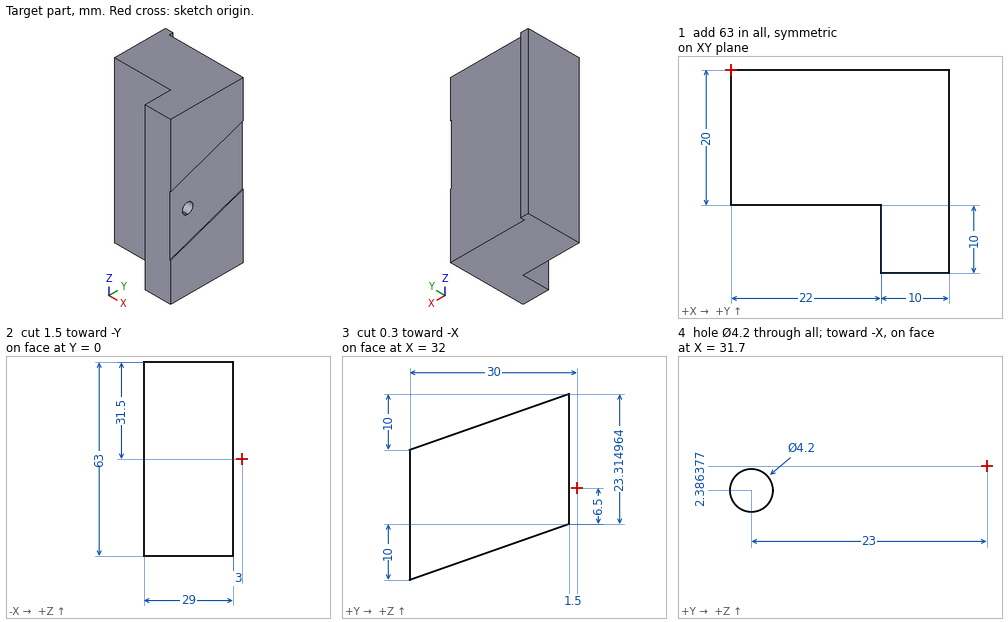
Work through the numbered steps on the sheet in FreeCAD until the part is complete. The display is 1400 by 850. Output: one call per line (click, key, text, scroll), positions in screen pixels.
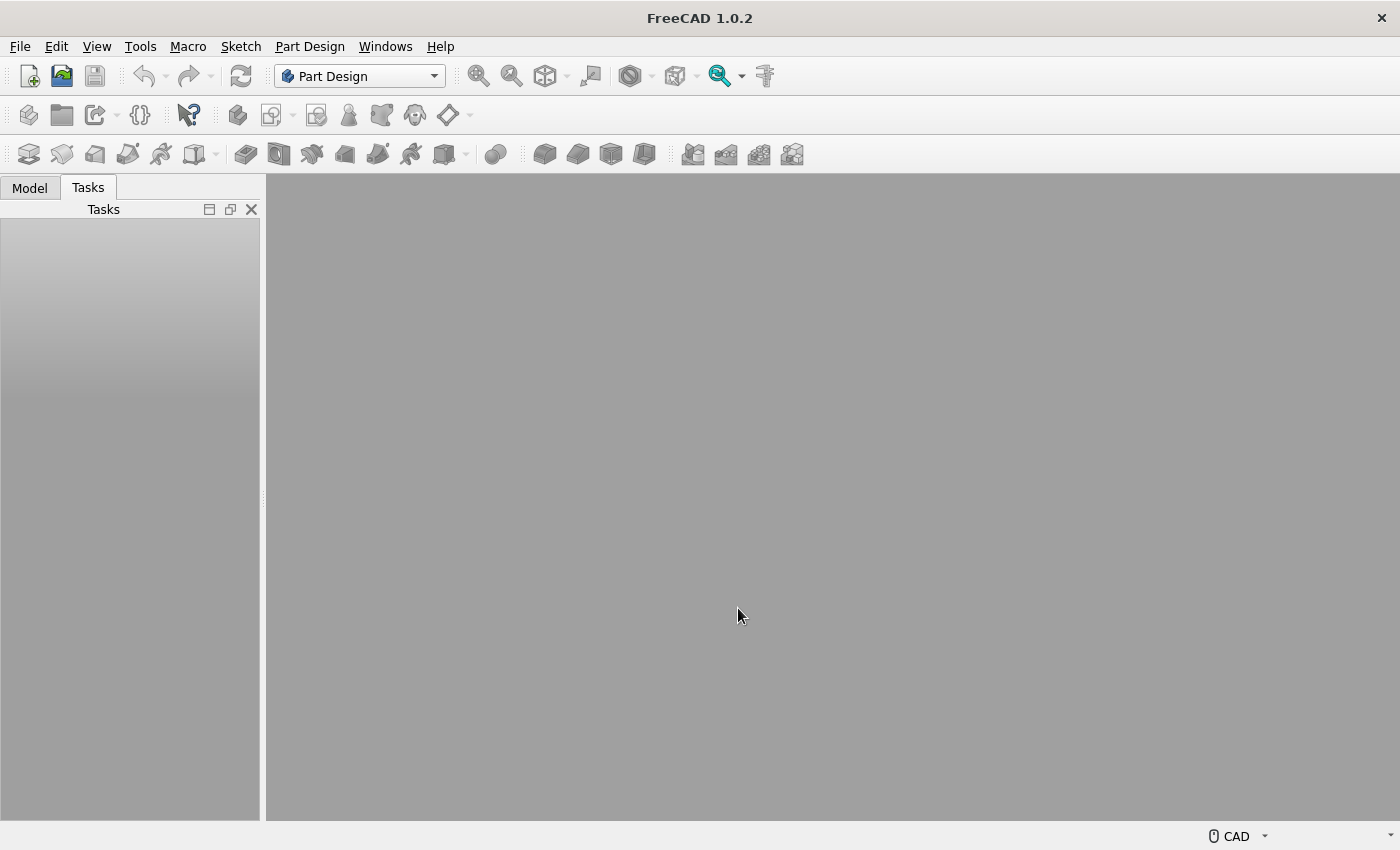
click(29, 76)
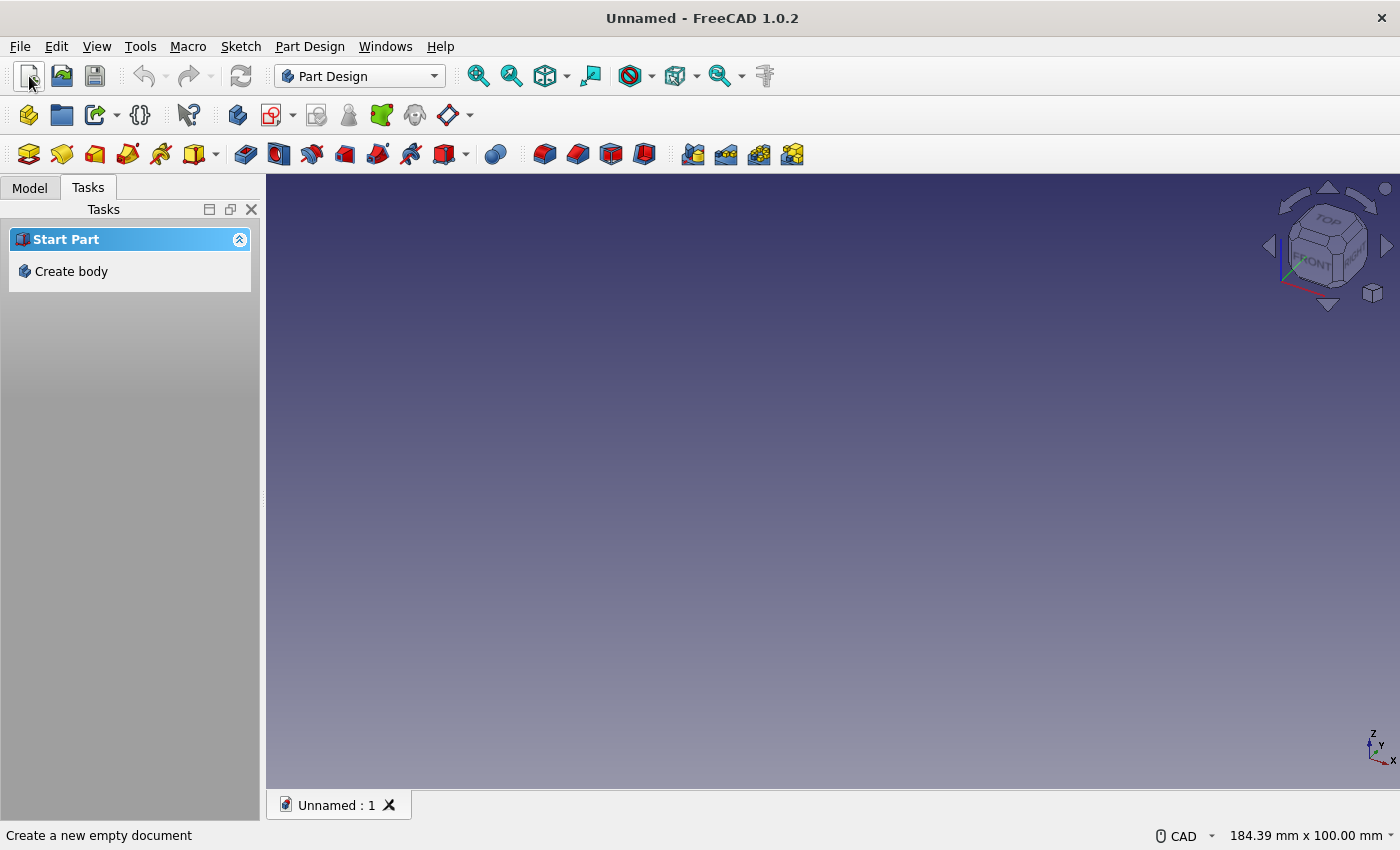
click(270, 116)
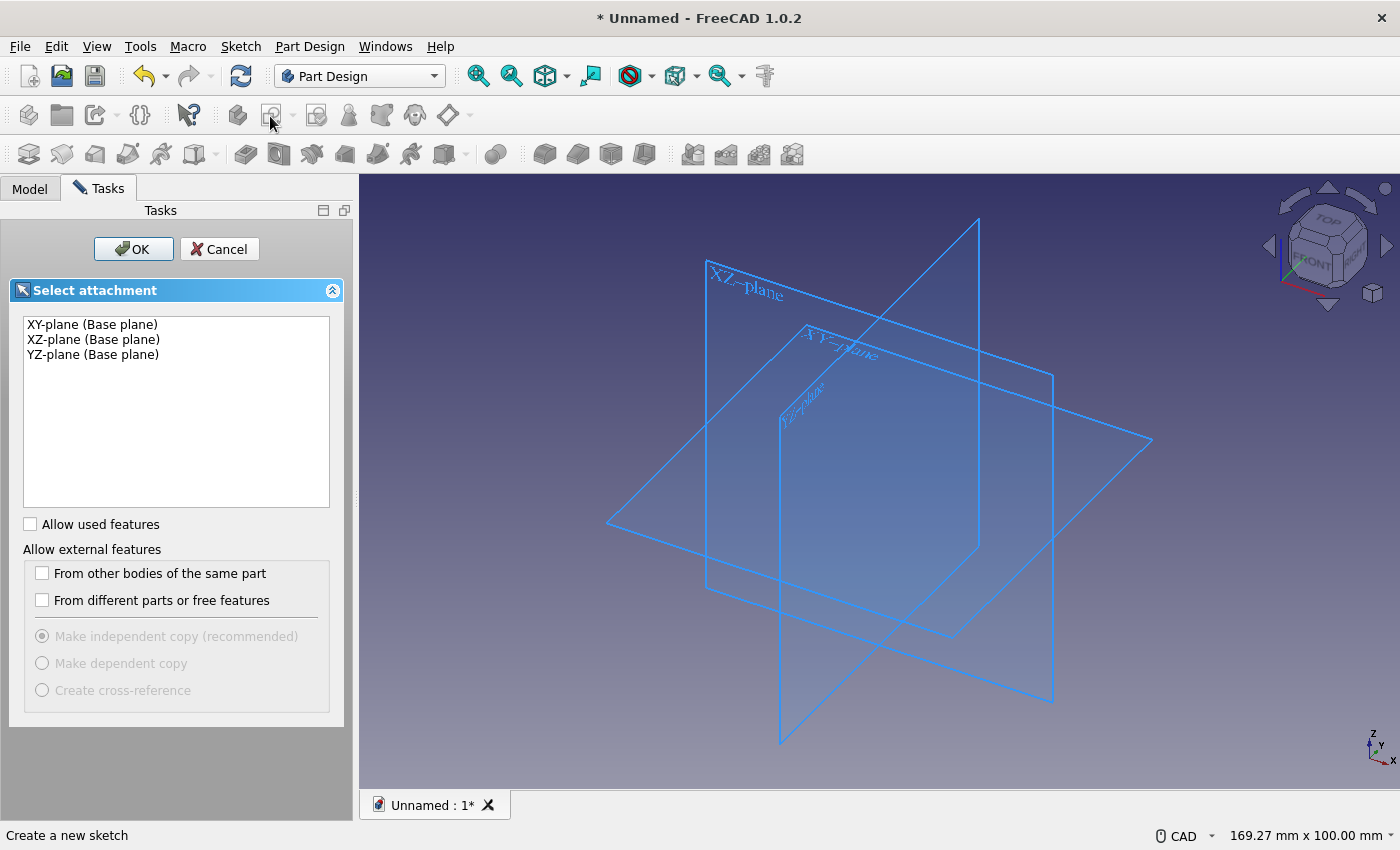
click(84, 324)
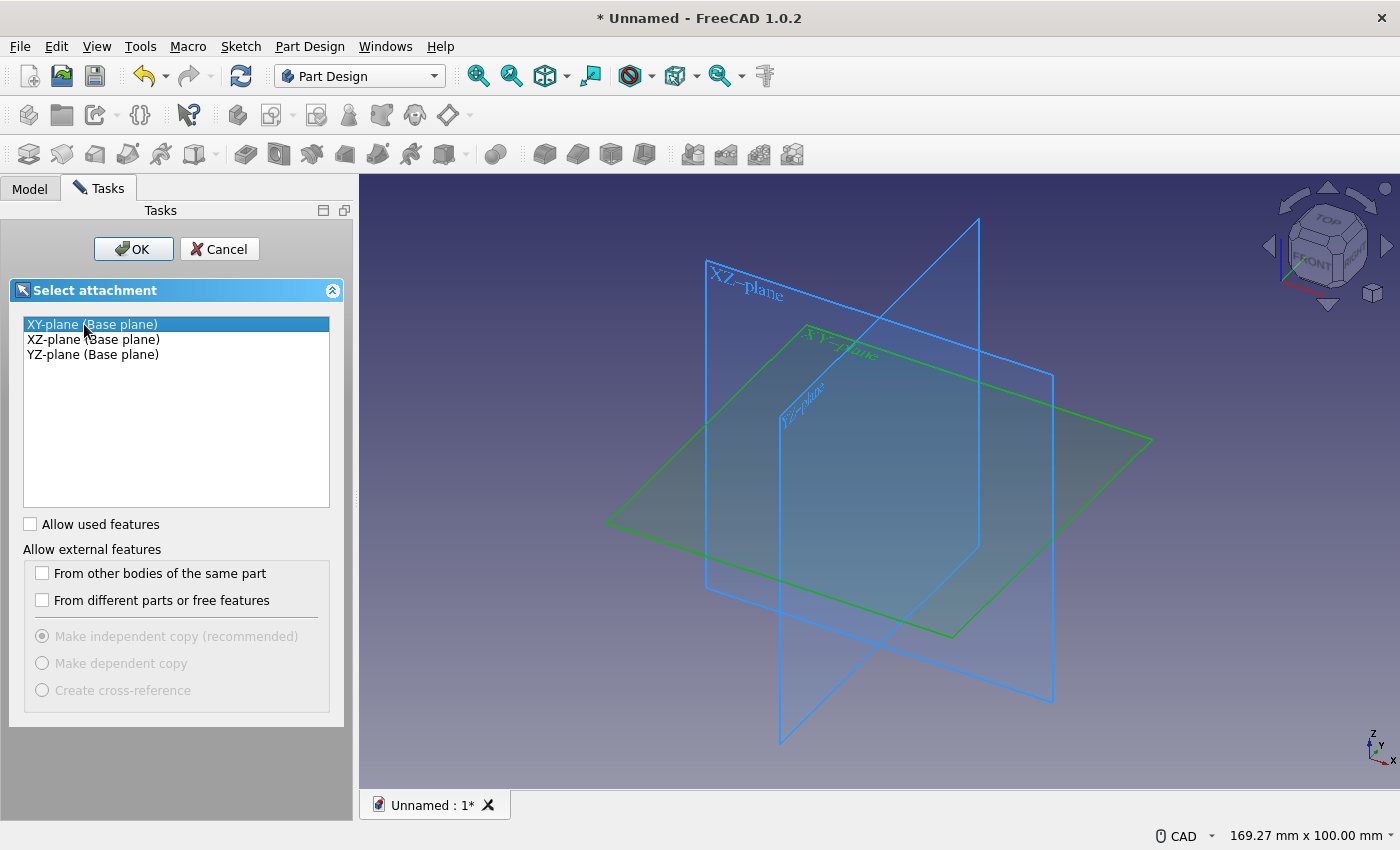
click(134, 249)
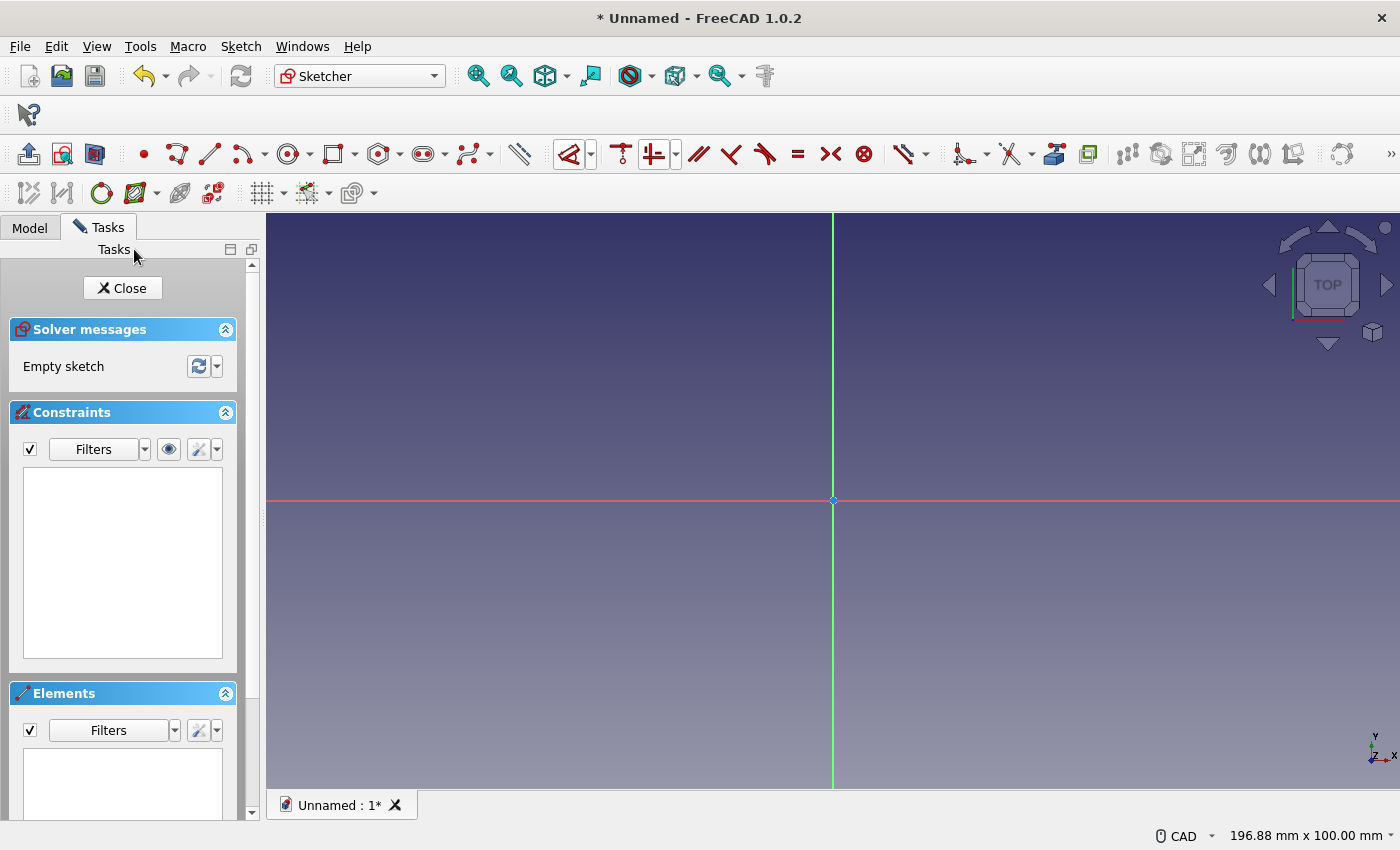
scroll(1056, 658, up, 4)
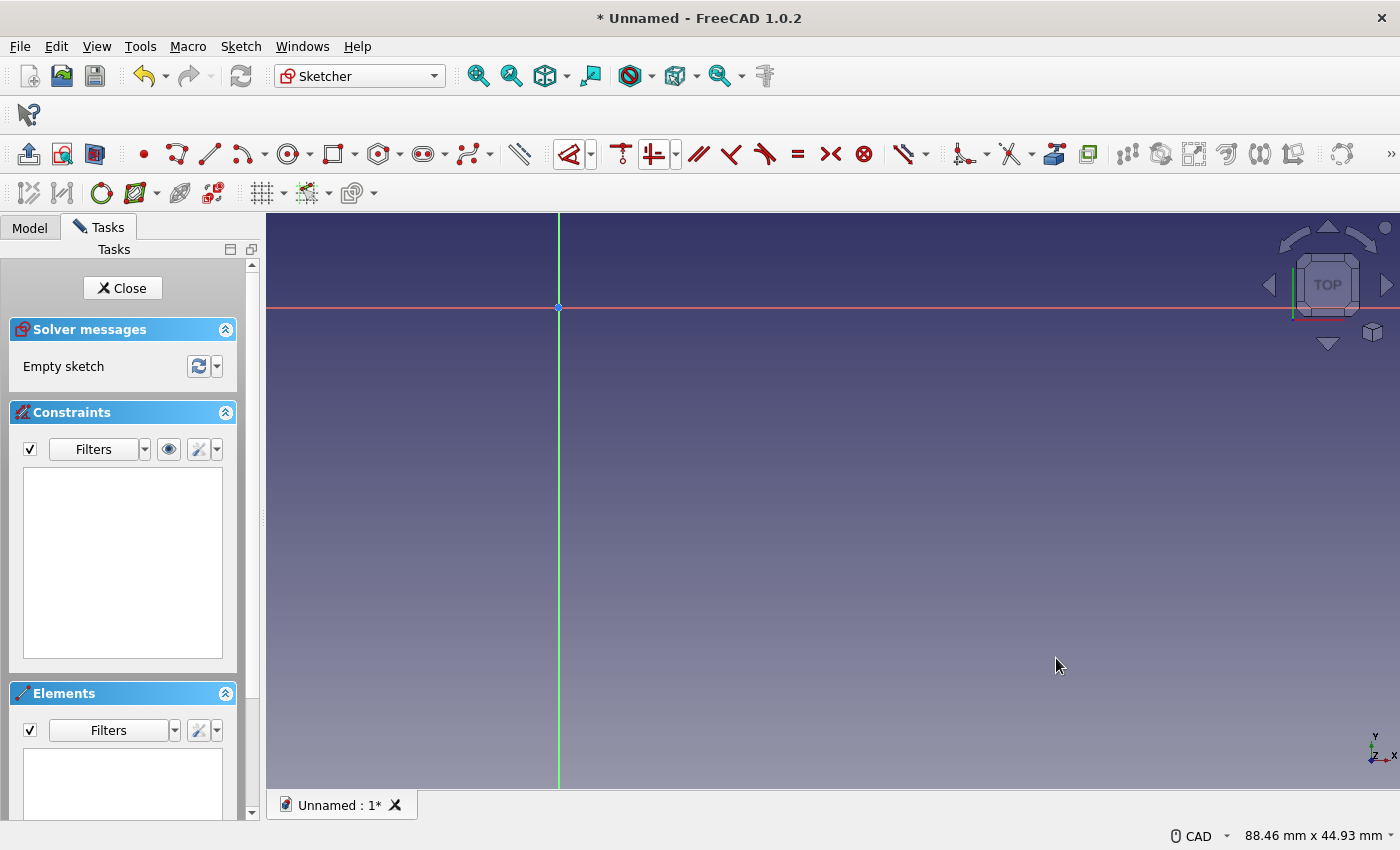
click(177, 154)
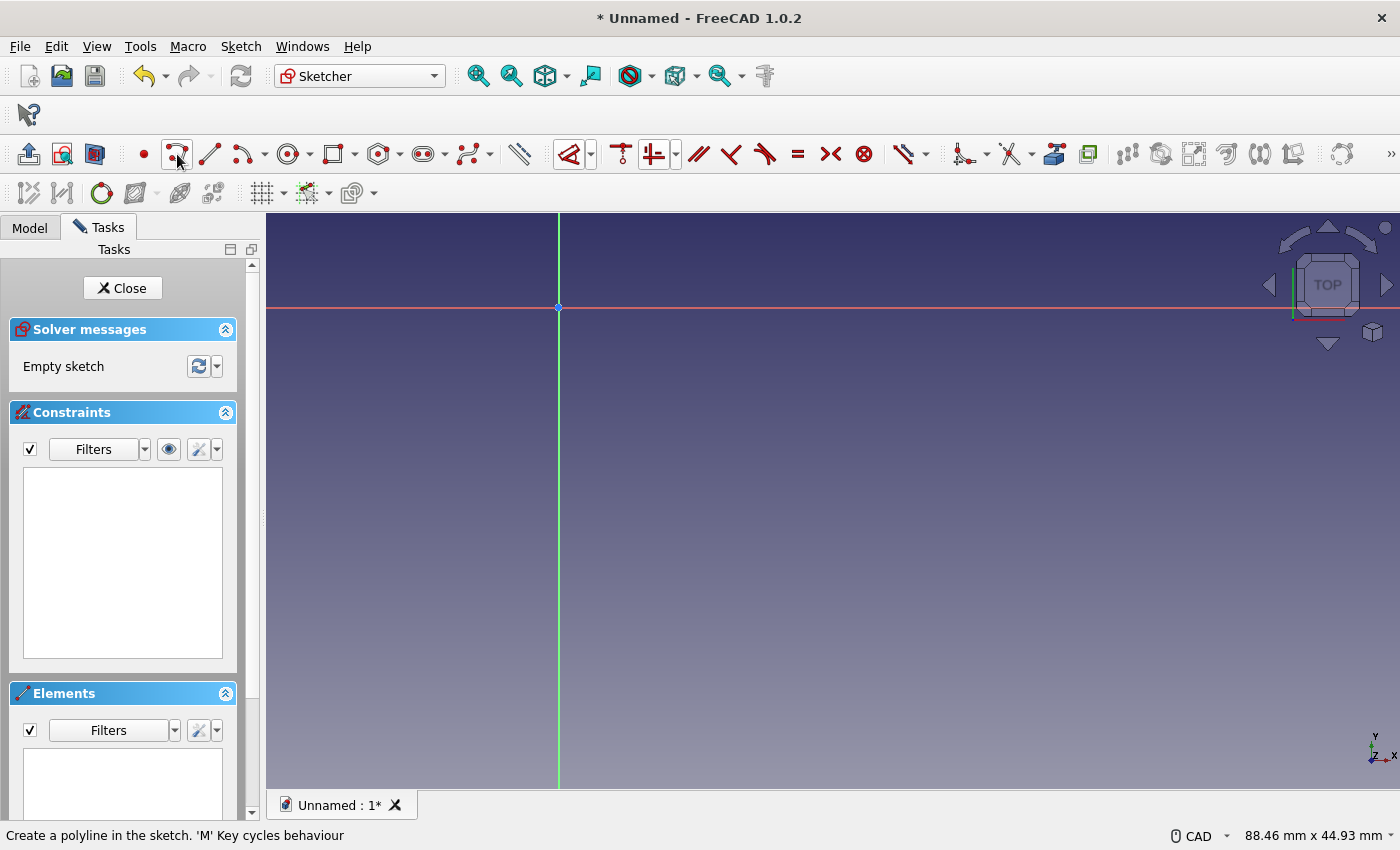
click(559, 308)
click(568, 564)
click(841, 564)
click(841, 692)
click(969, 692)
click(969, 317)
click(559, 308)
key(Escape)
key(Escape)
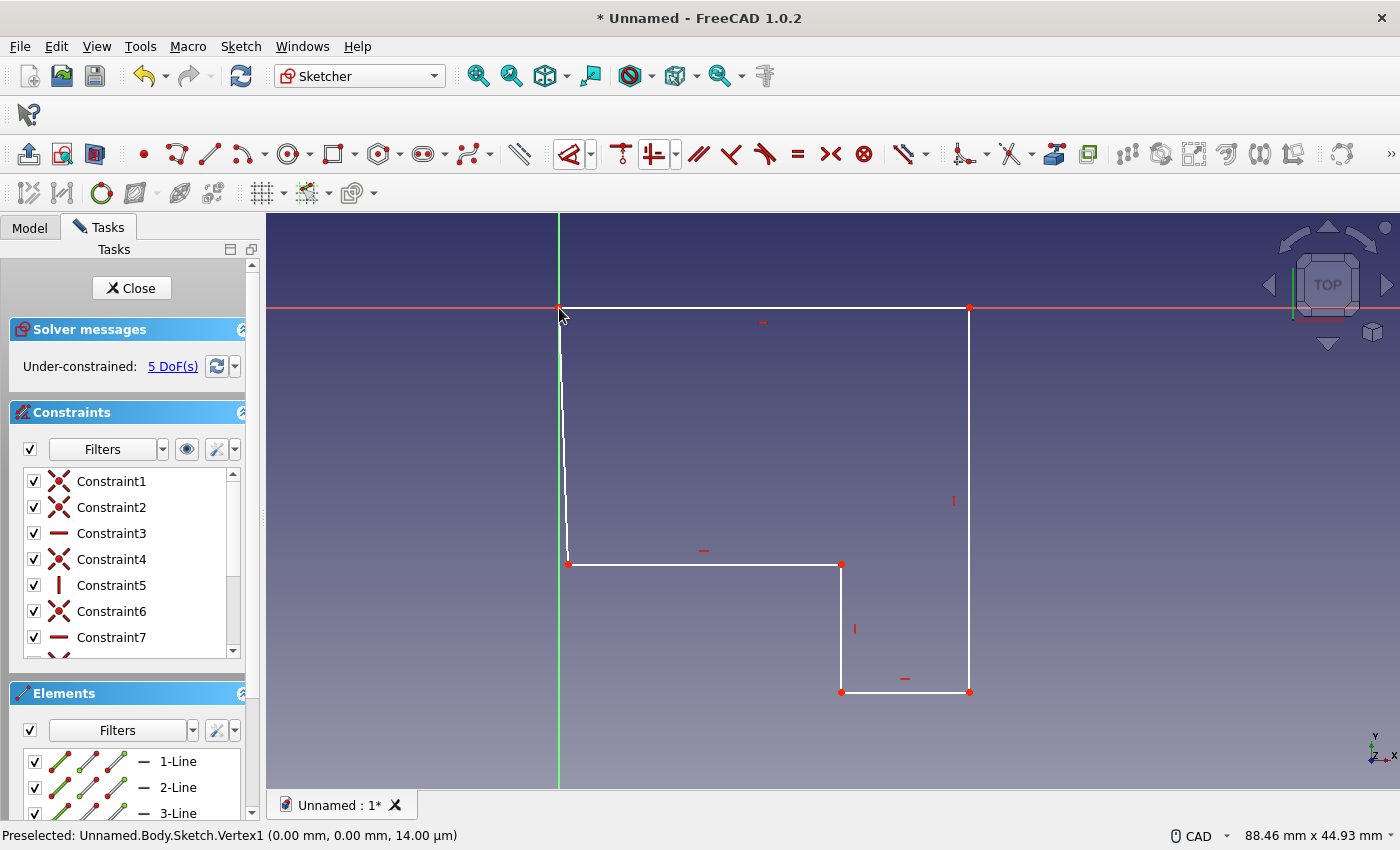
click(562, 385)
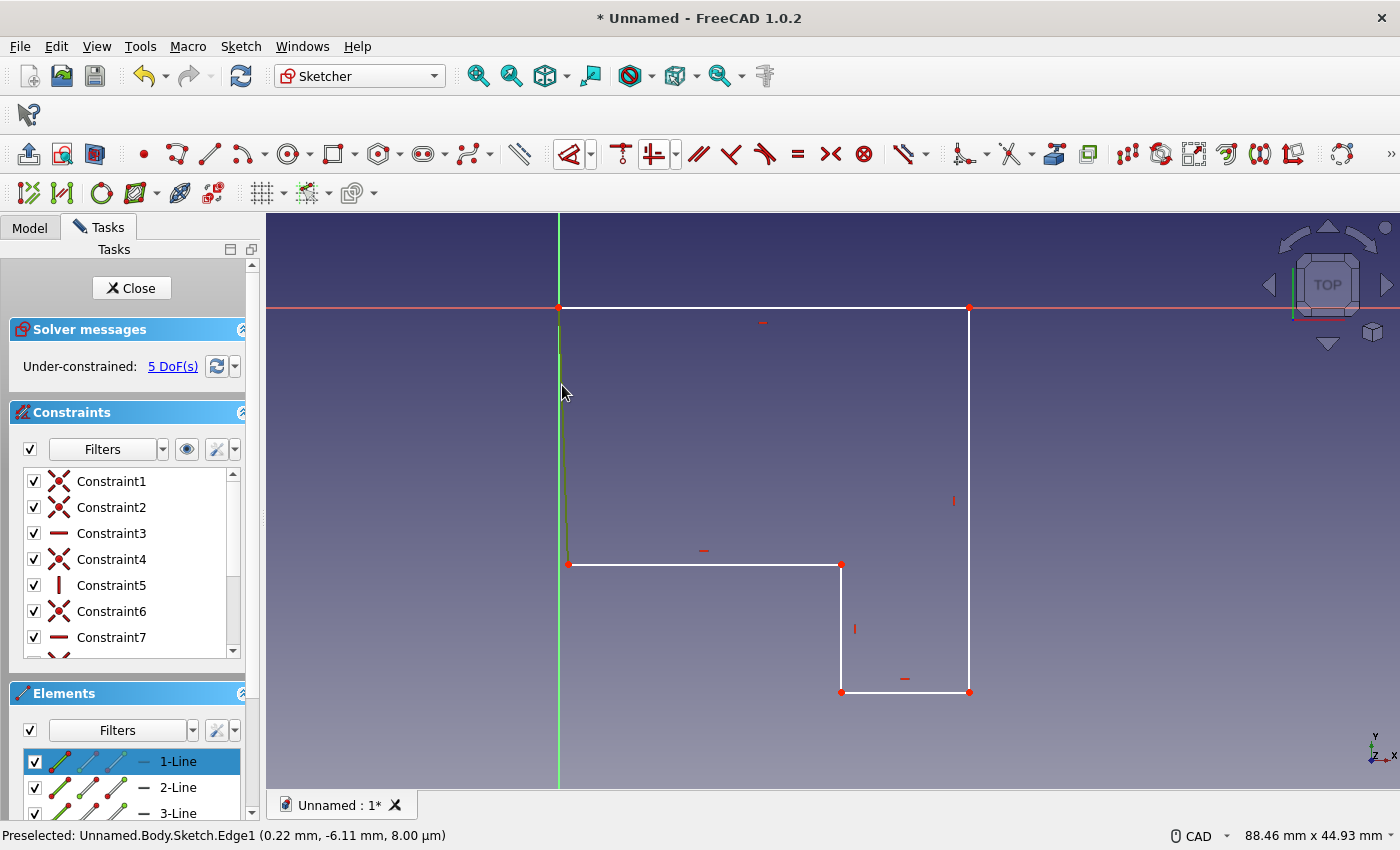
click(676, 154)